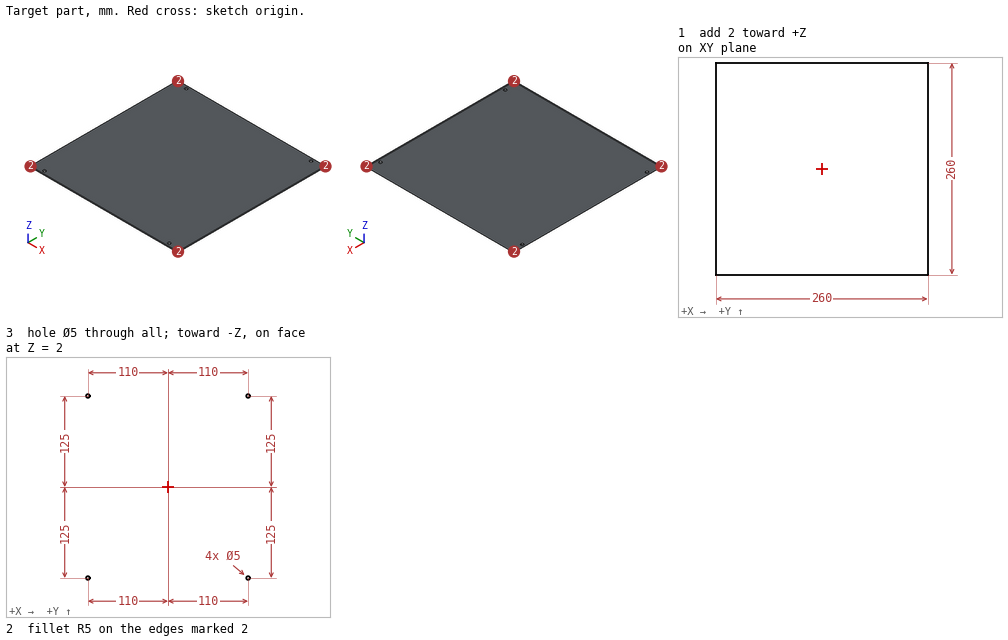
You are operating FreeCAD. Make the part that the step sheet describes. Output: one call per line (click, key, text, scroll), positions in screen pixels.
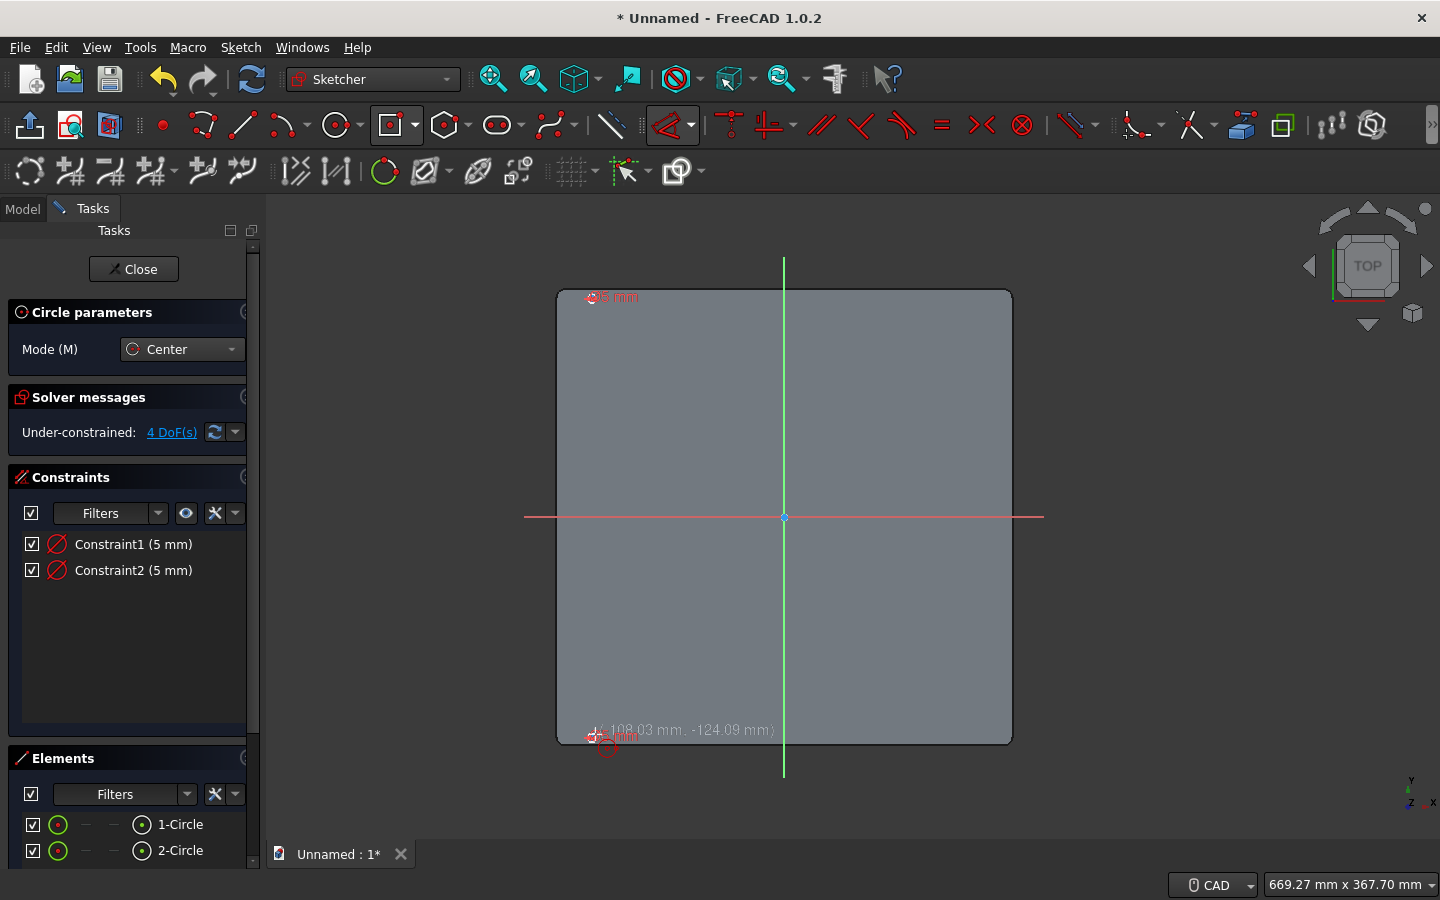
scroll(977, 737, up, 9)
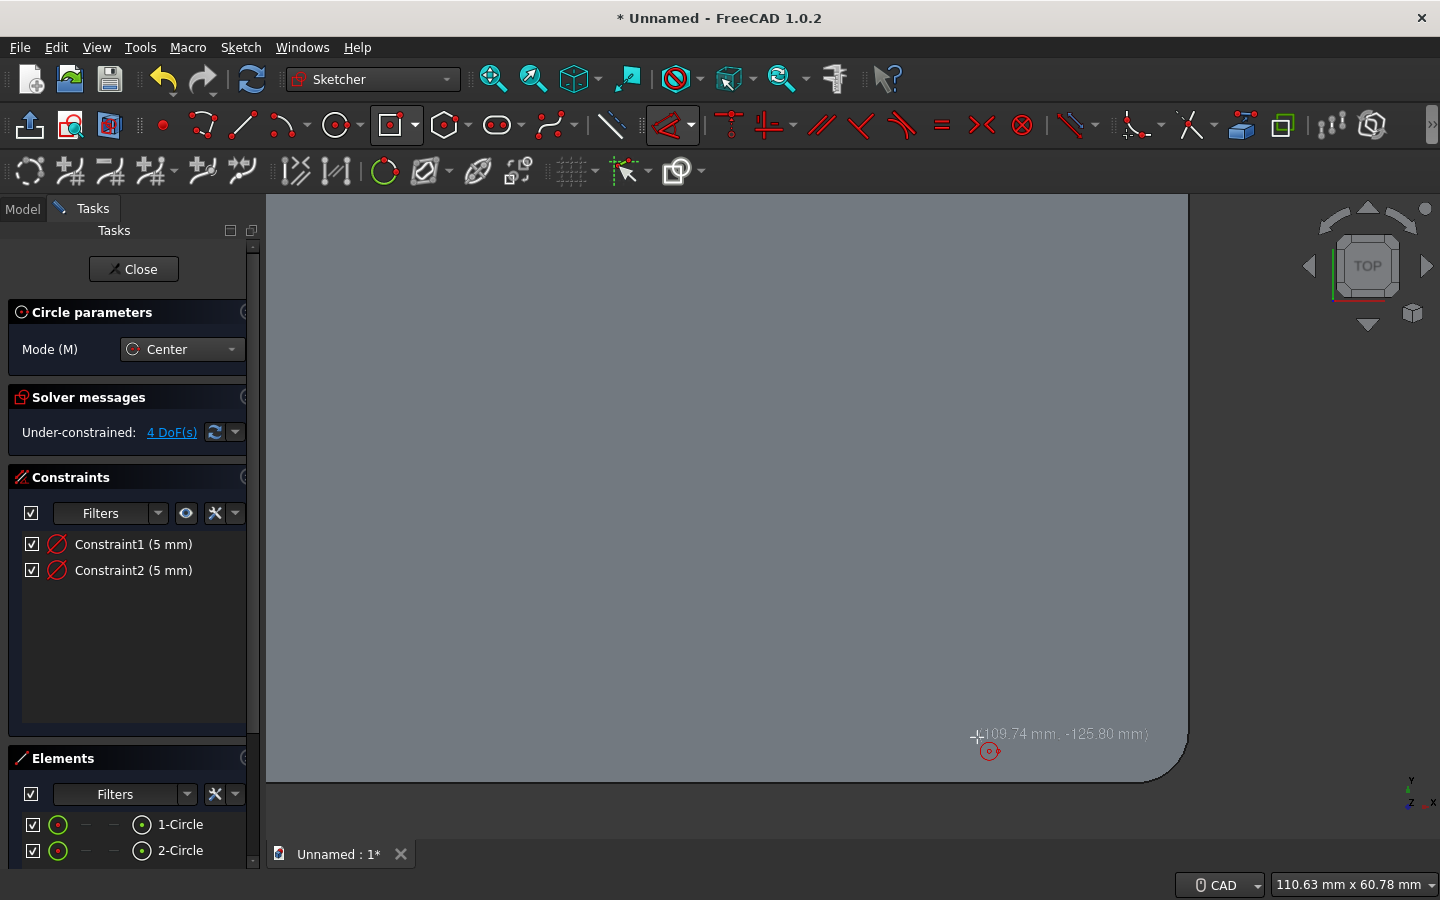
scroll(978, 737, down, 9)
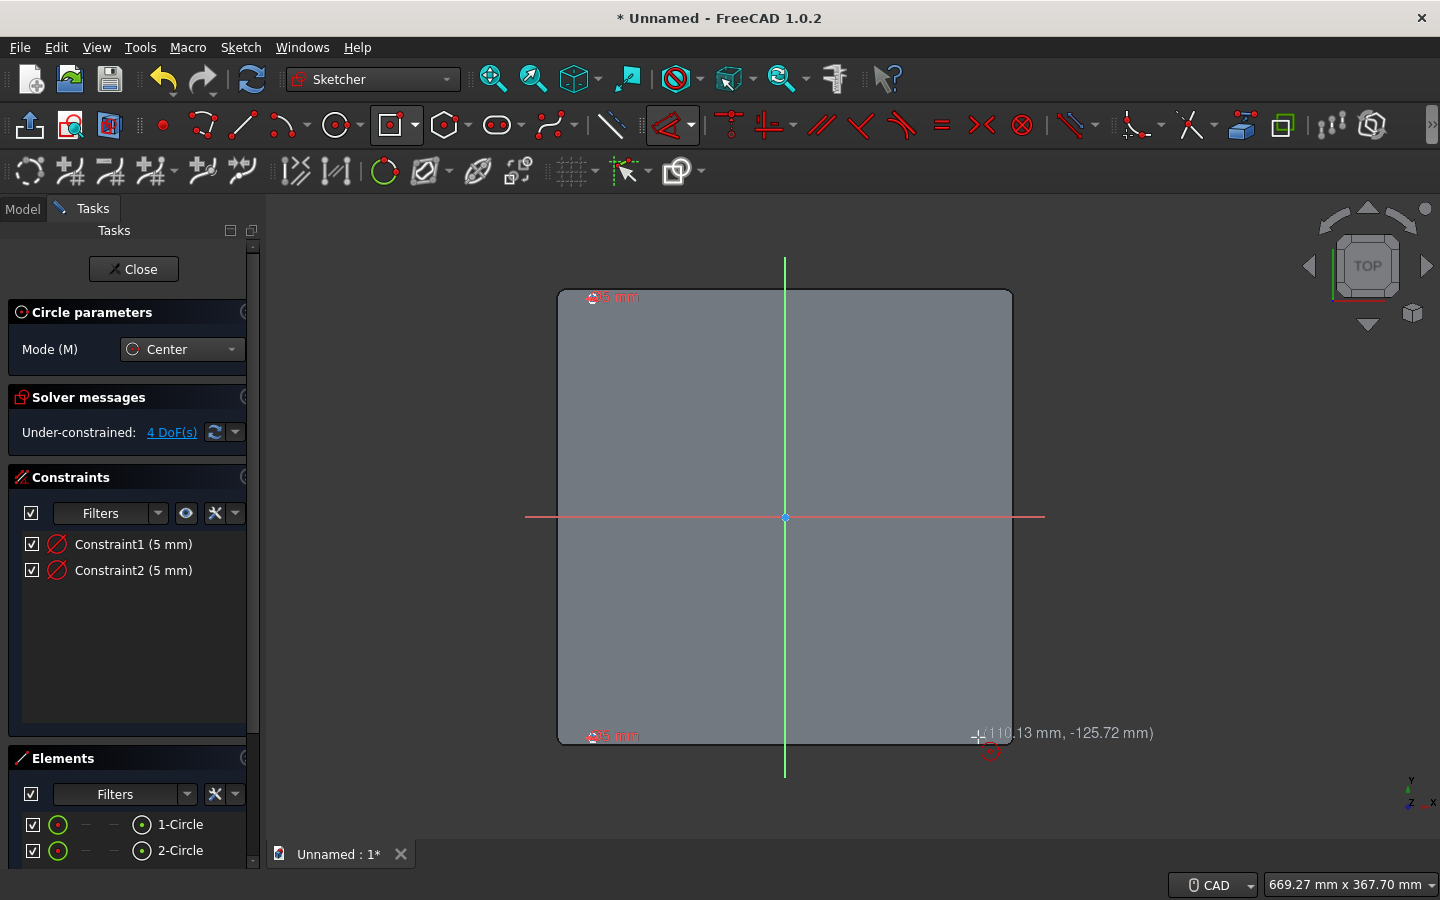
click(978, 737)
move(981, 734)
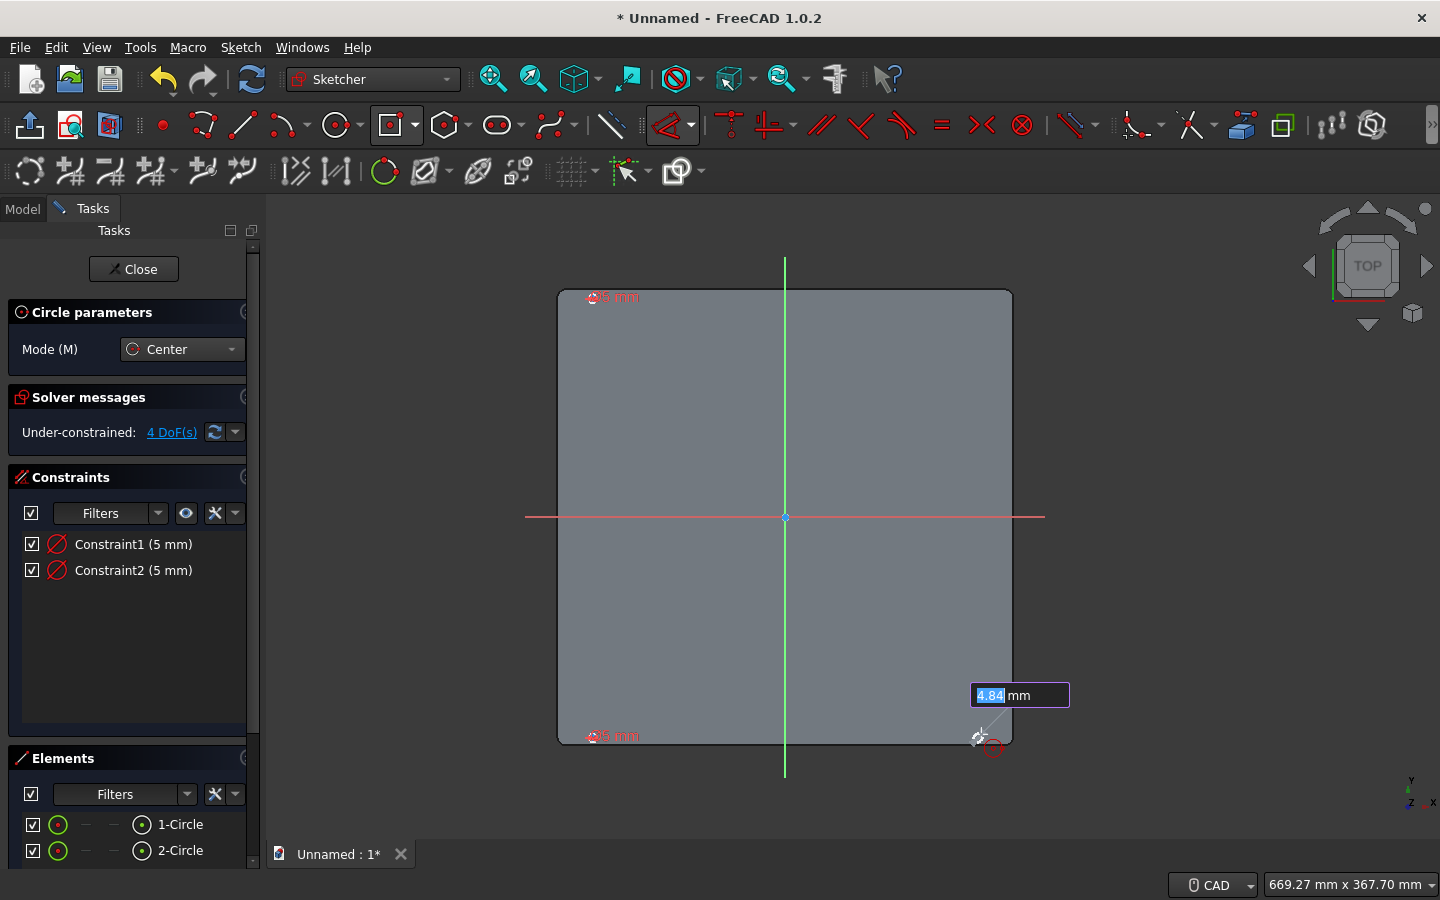
text(5)
key(Return)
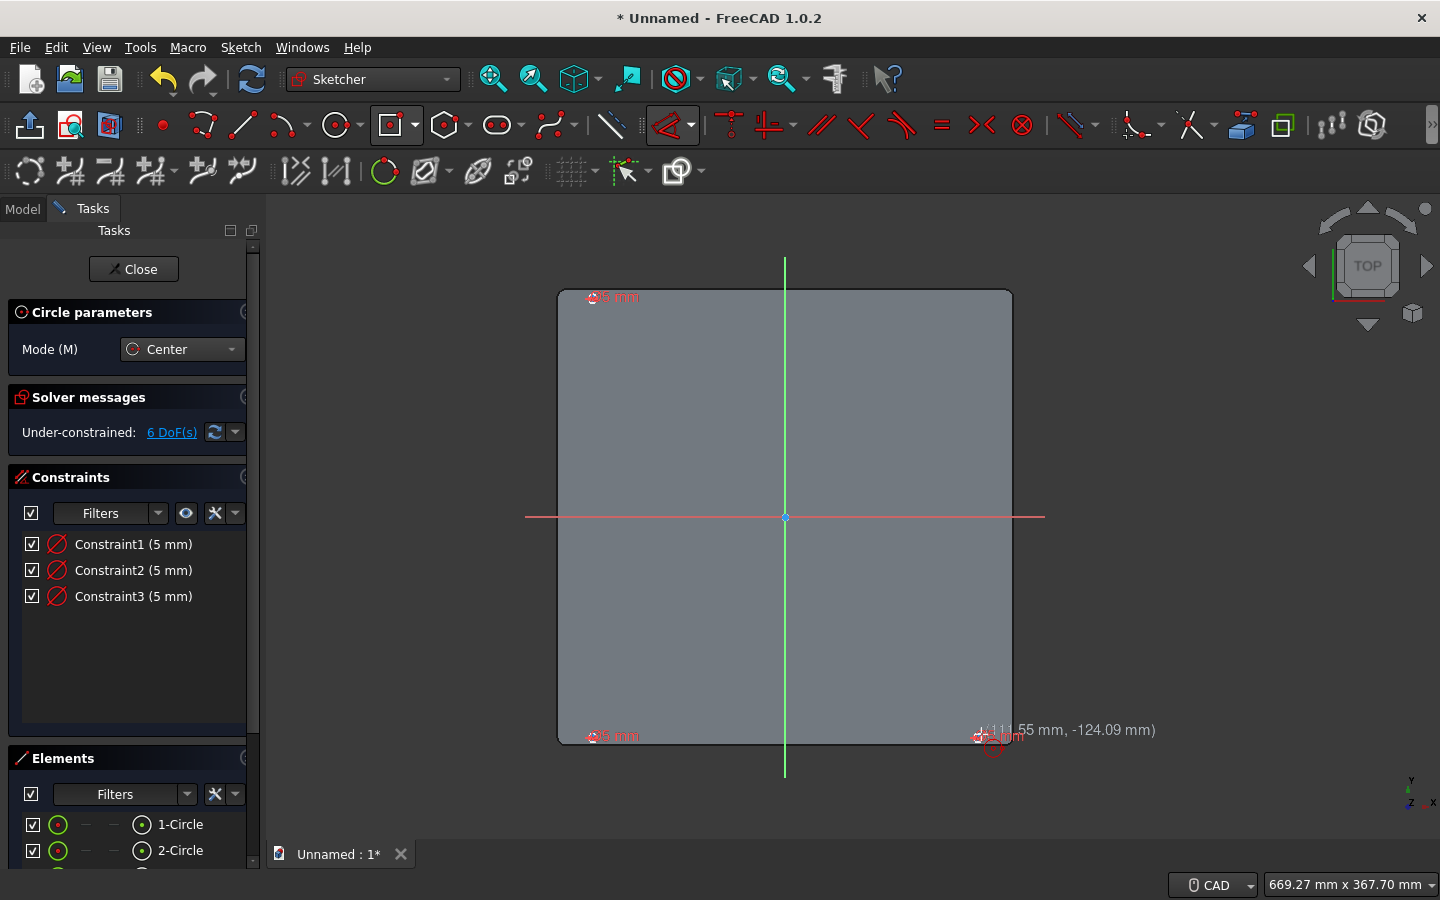
scroll(978, 298, up, 9)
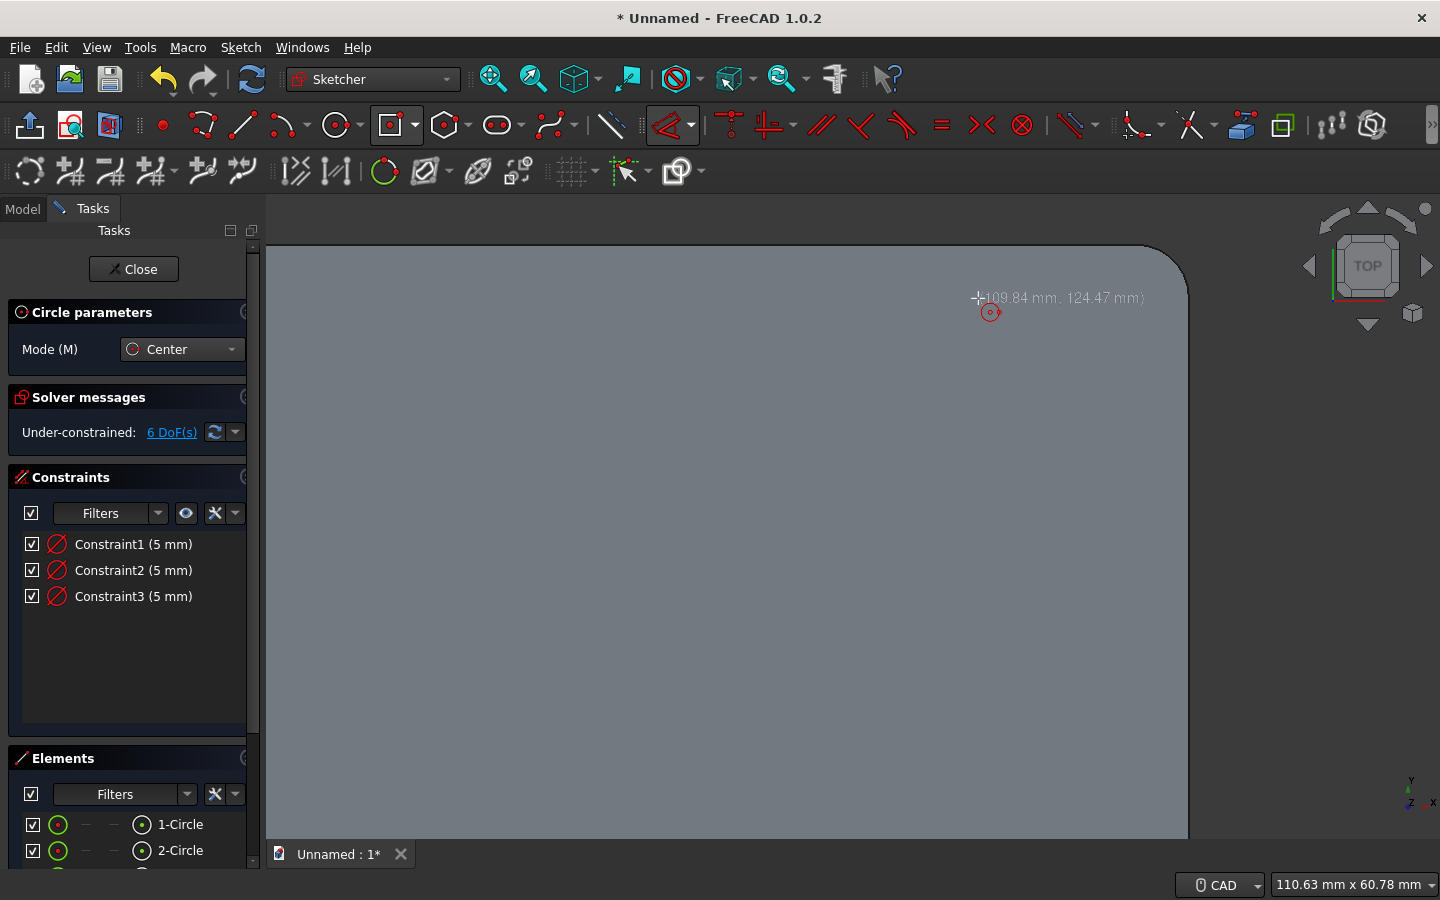
scroll(978, 297, down, 9)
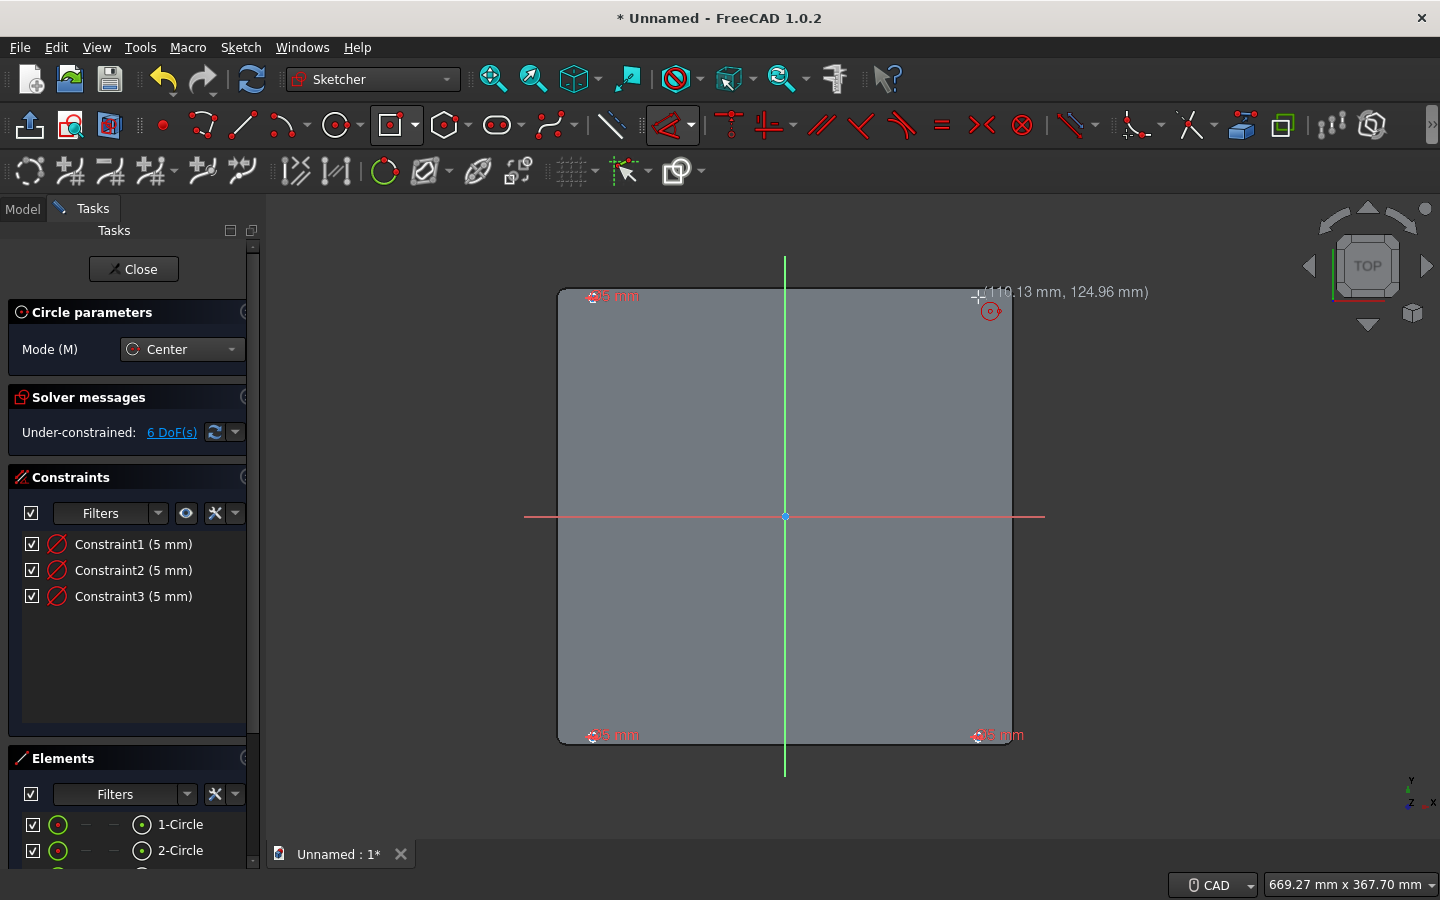
click(978, 297)
move(981, 294)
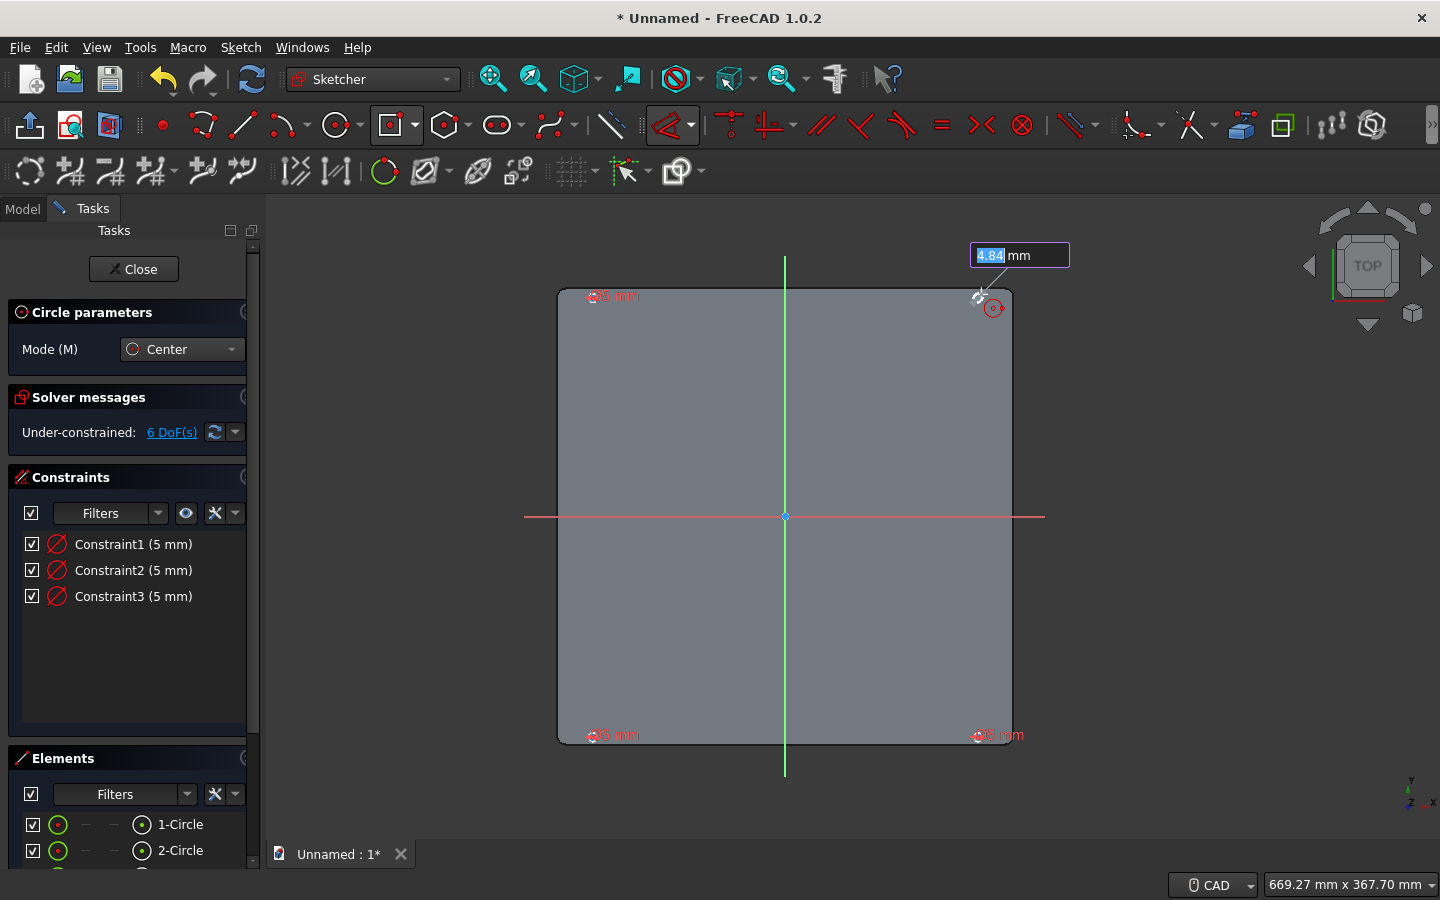
text(5)
key(Return)
key(Escape)